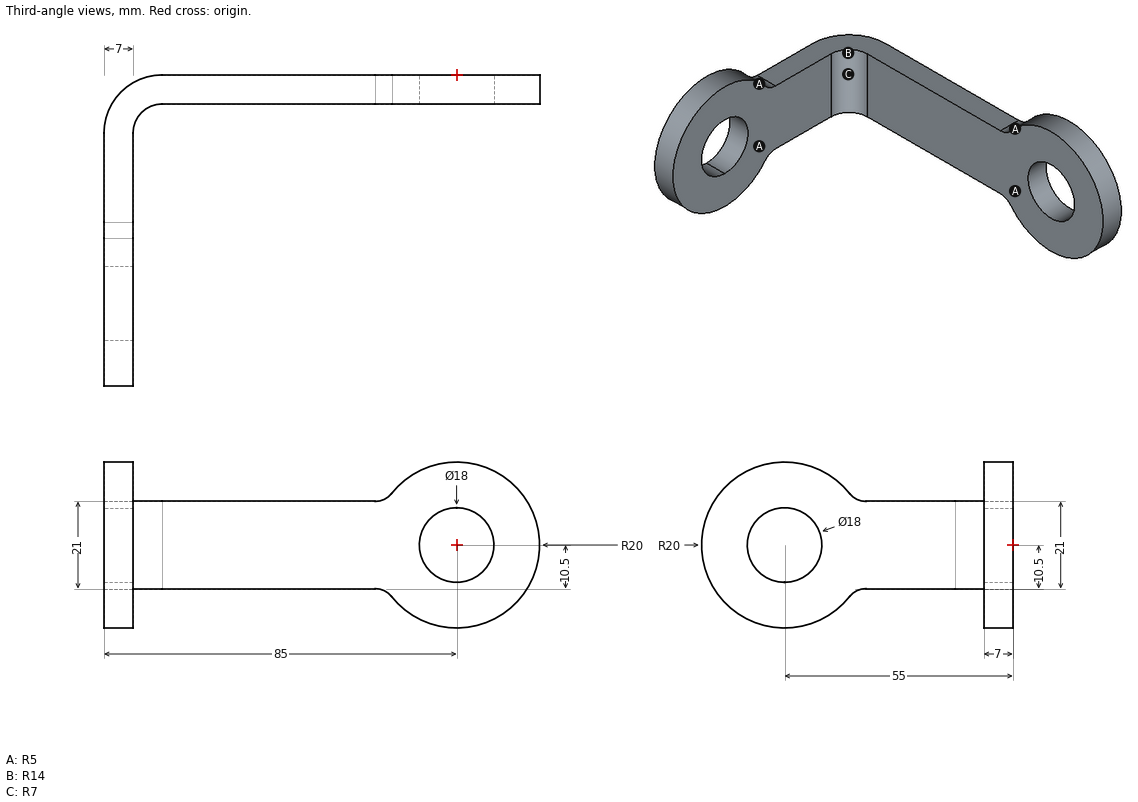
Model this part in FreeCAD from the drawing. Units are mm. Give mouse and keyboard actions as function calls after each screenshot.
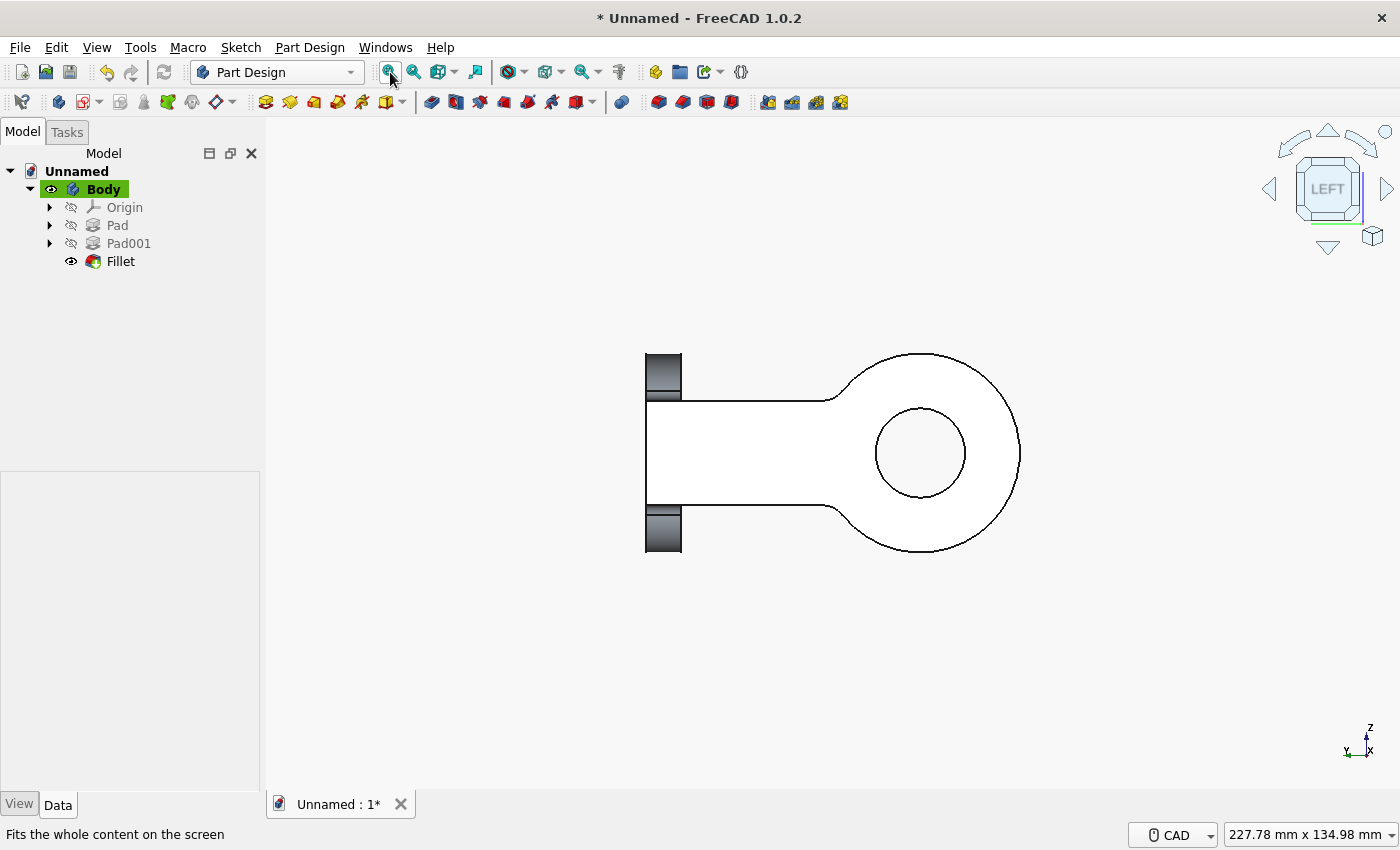
click(646, 452)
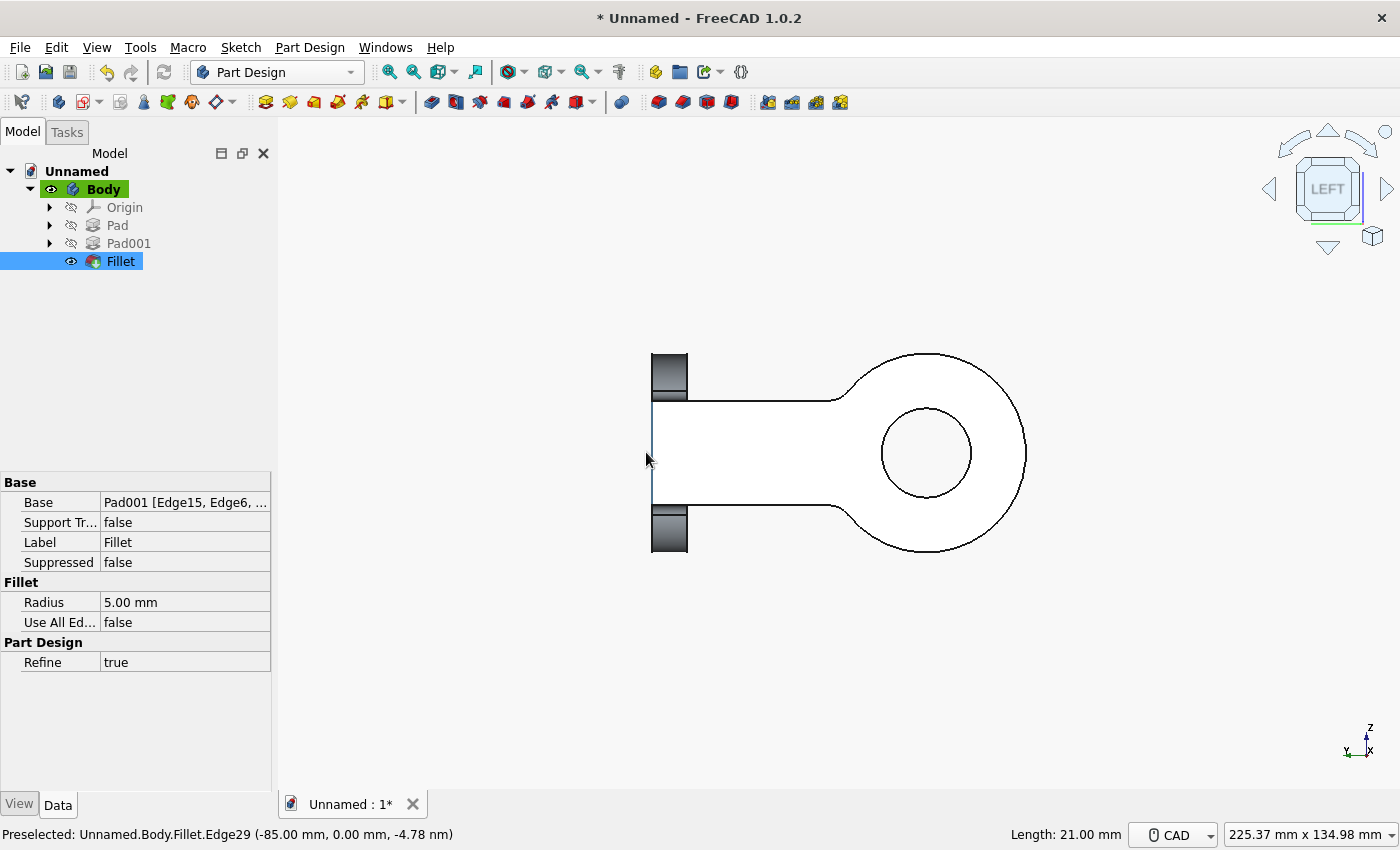
click(660, 102)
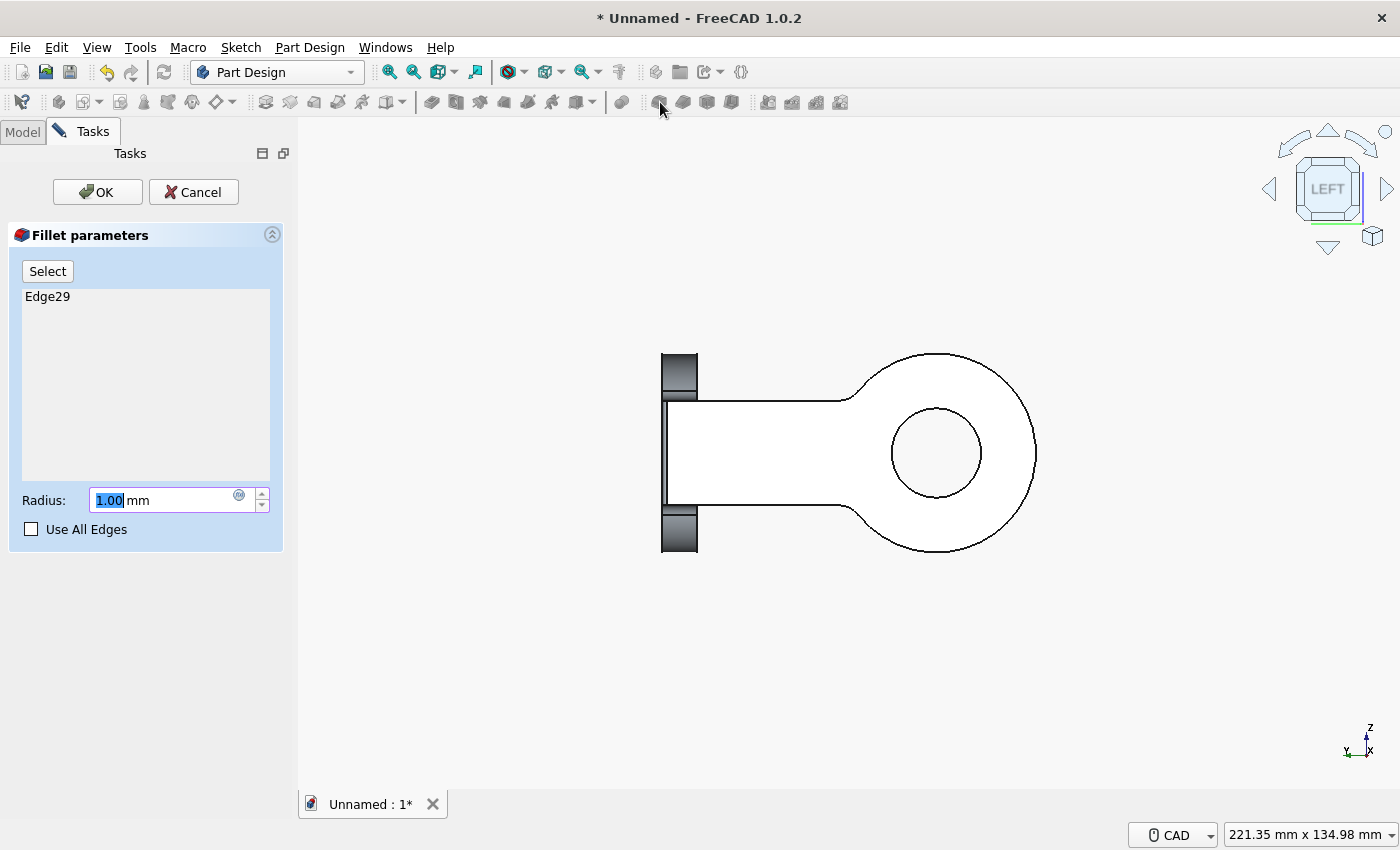
text(14)
key(Tab)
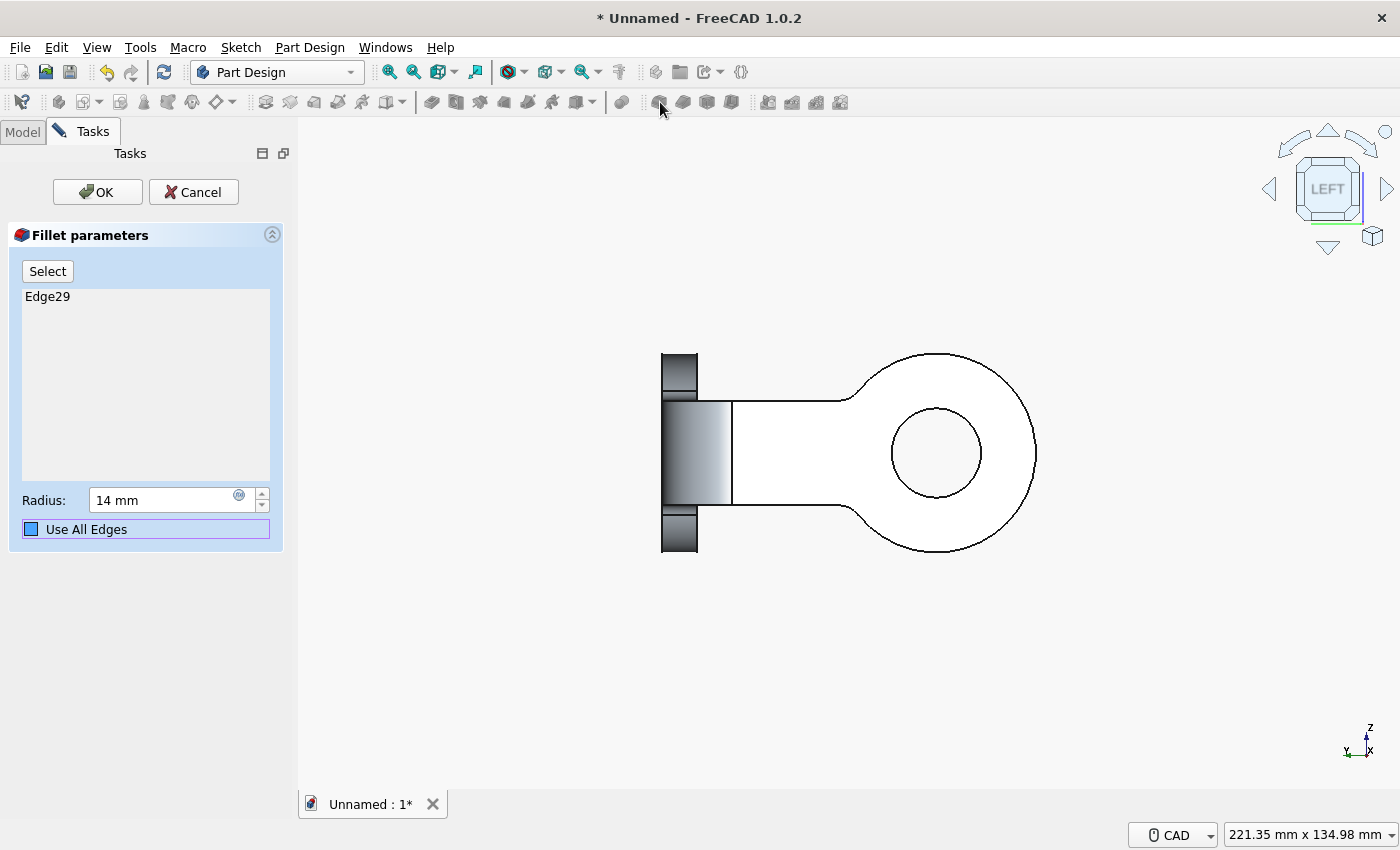
click(98, 192)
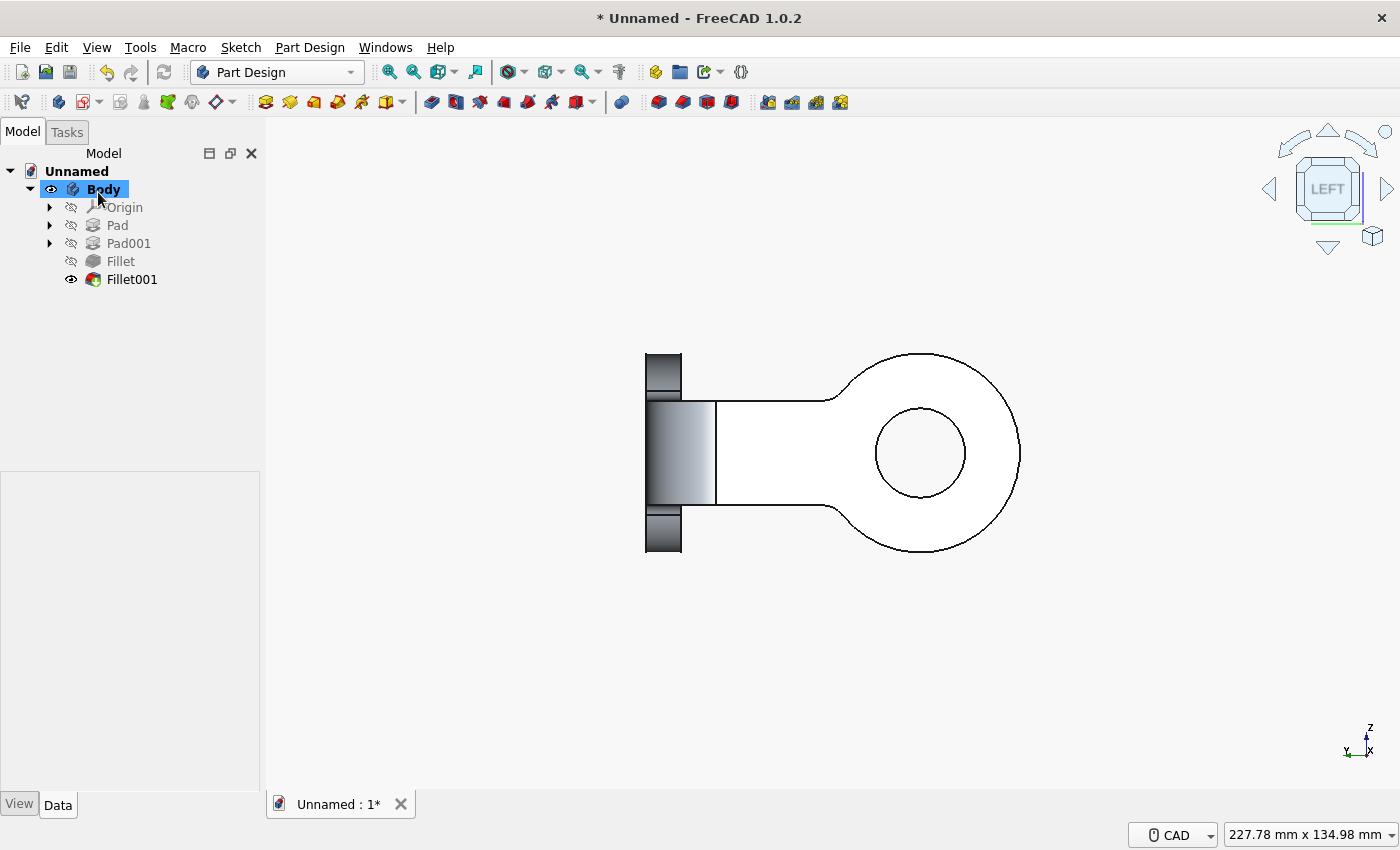
click(390, 72)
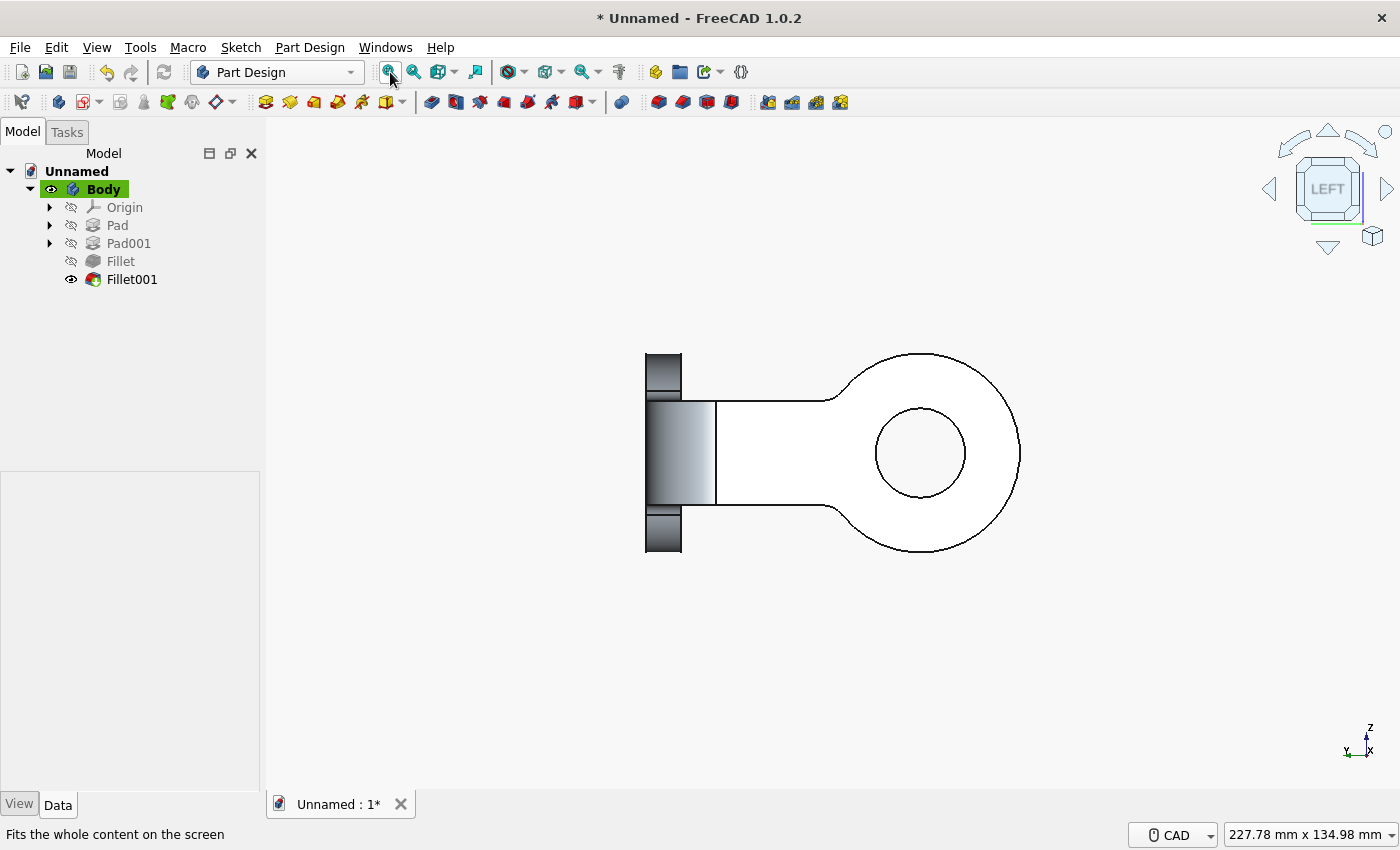
key(0)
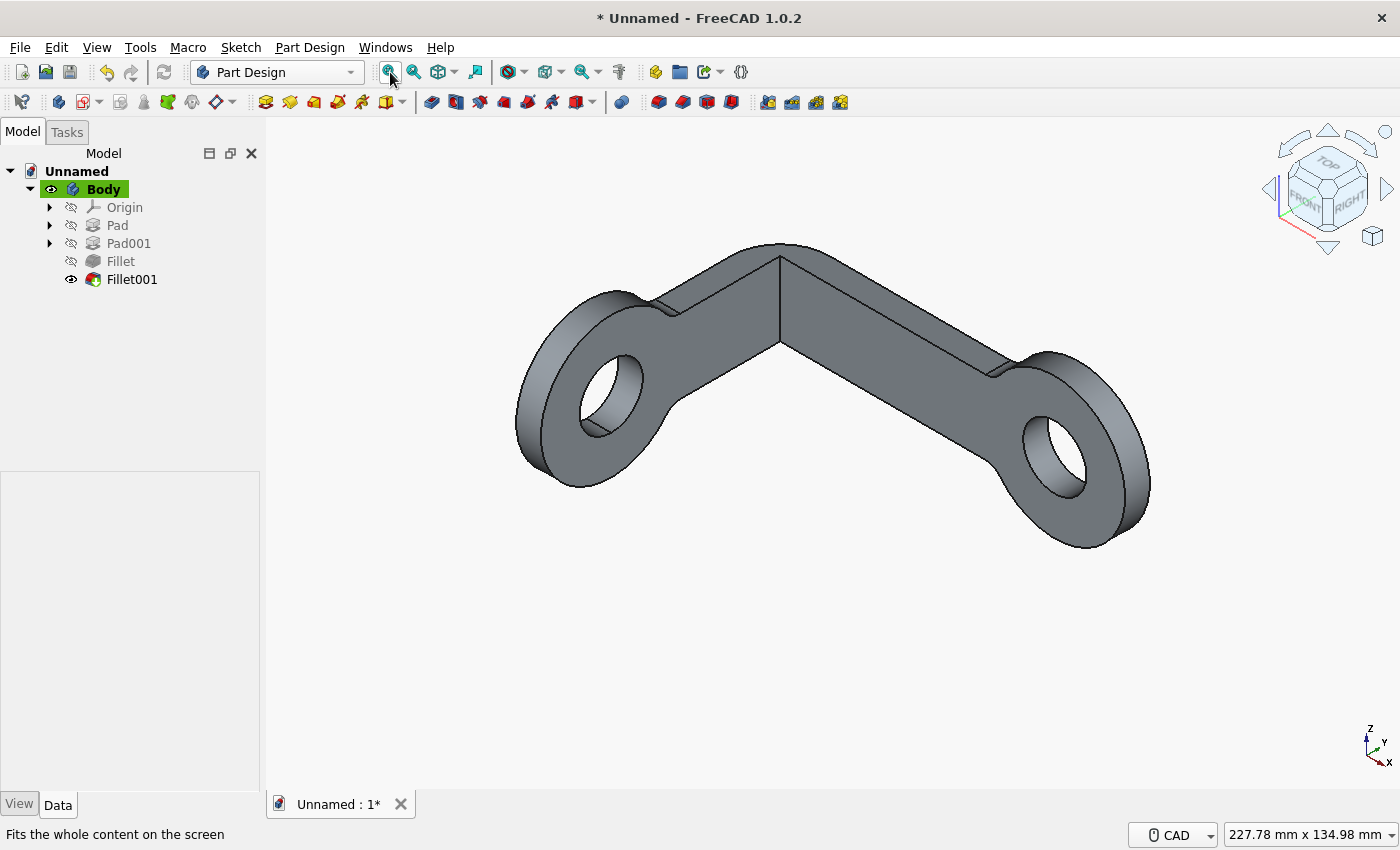
key(2)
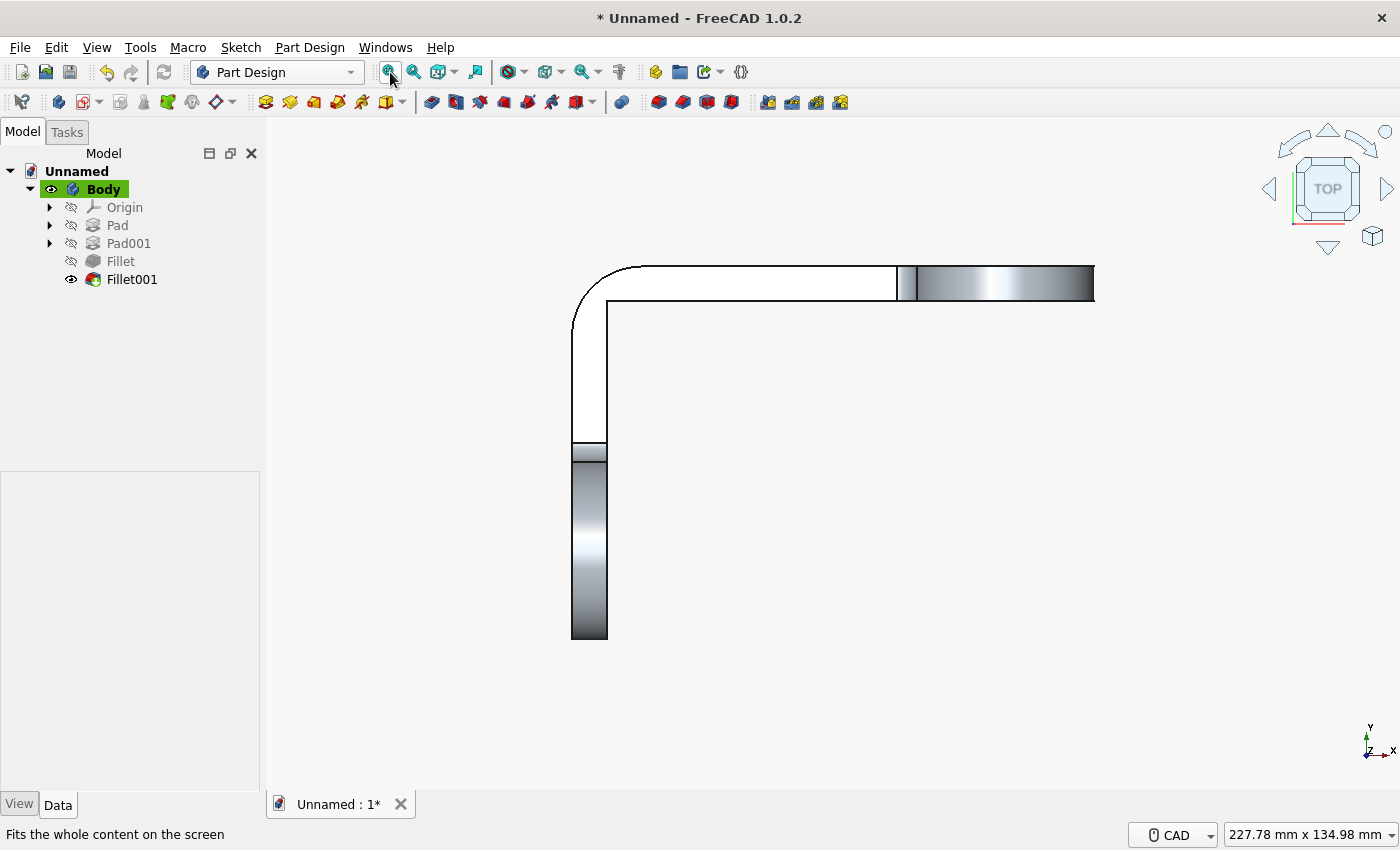
key(1)